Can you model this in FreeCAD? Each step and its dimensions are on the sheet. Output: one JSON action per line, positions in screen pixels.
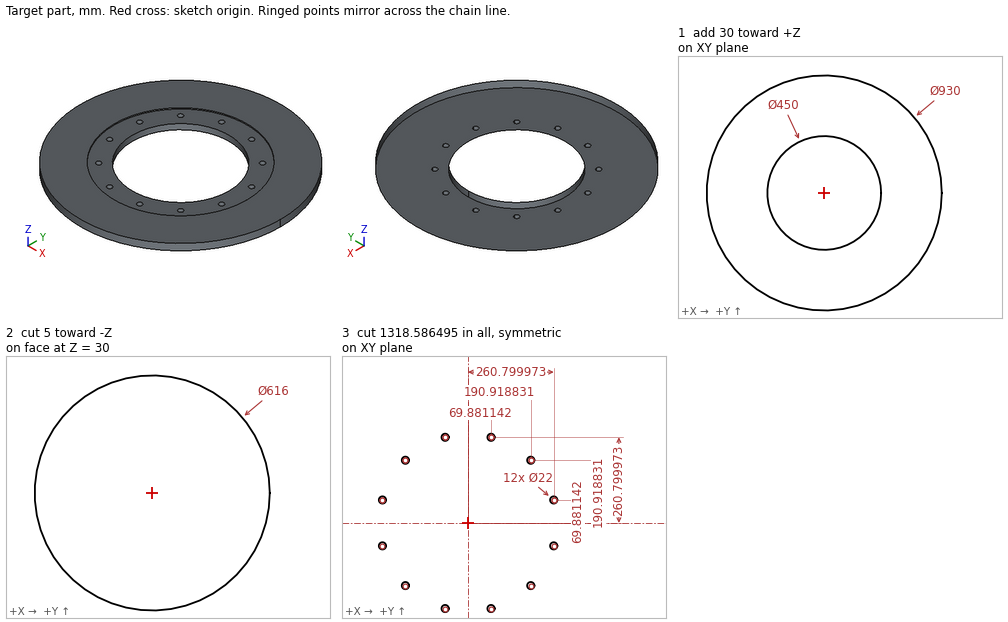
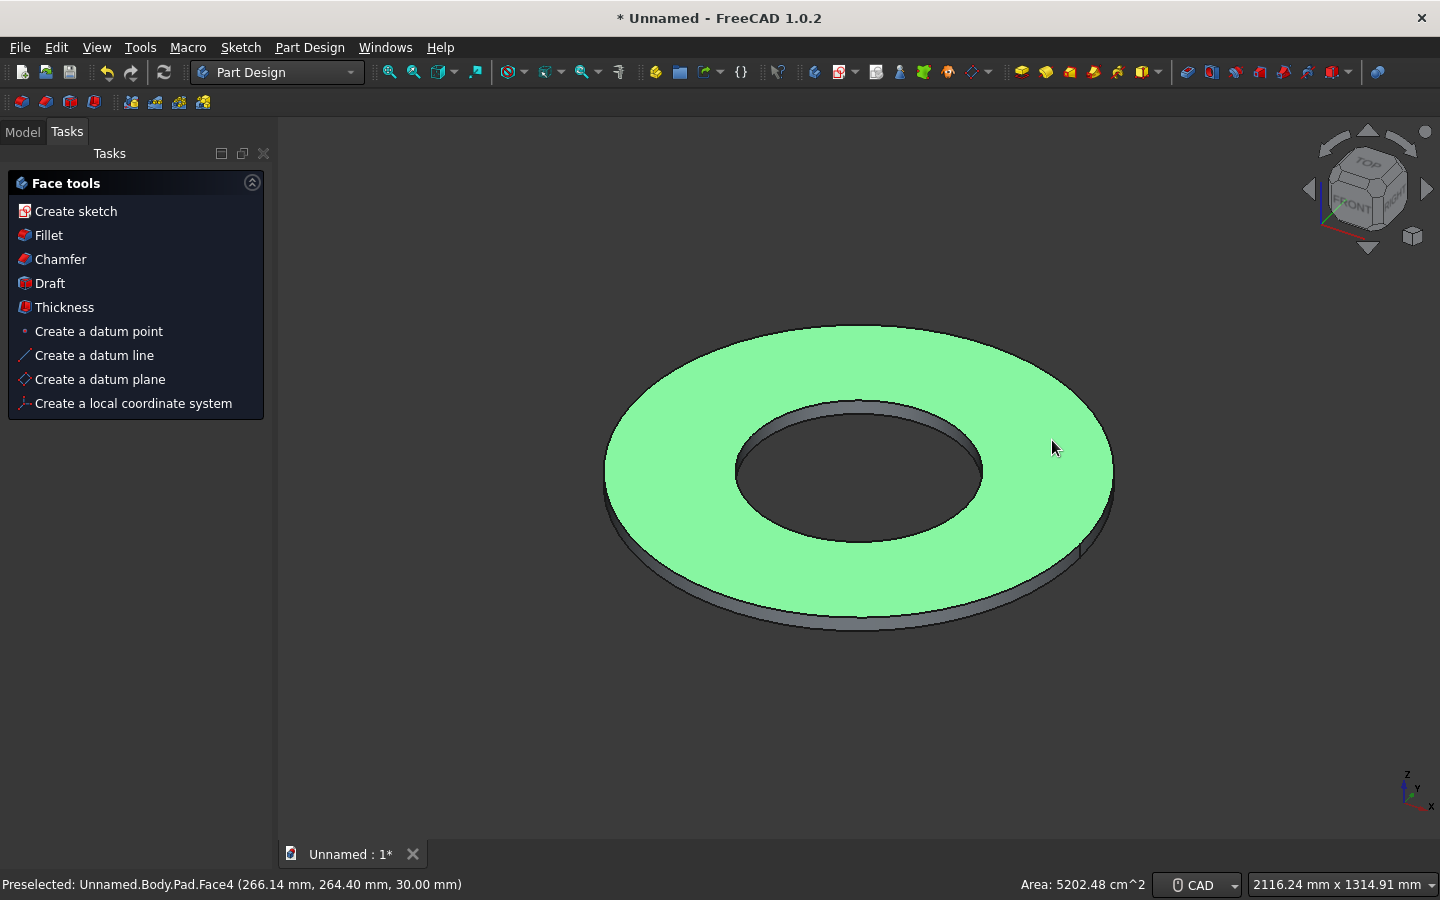
{"action": "left_click", "coordinate": [840, 72]}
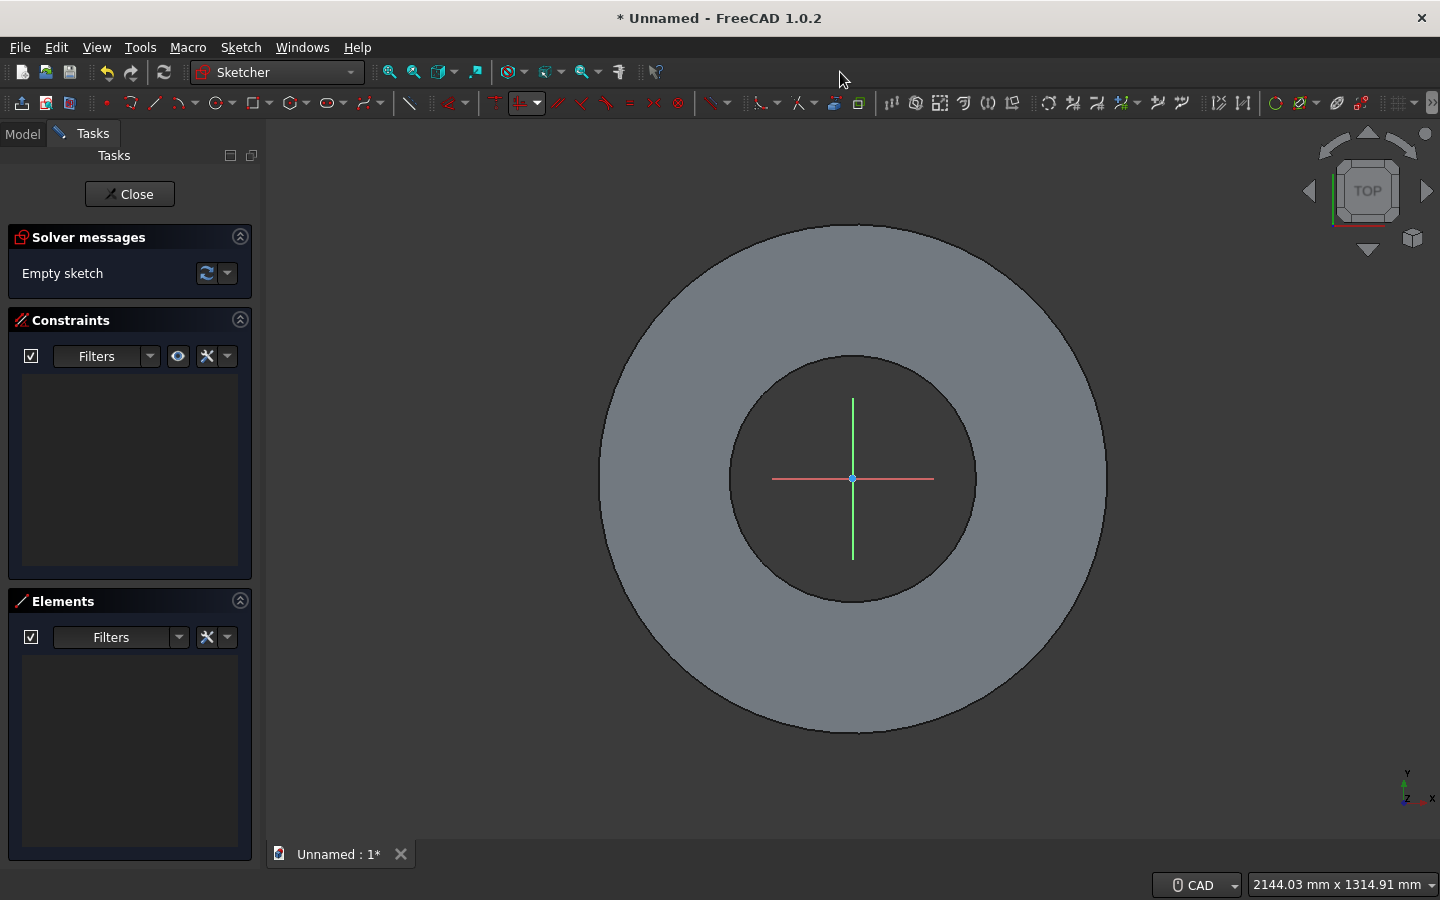
{"action": "scroll", "coordinate": [992, 479], "scroll_direction": "up", "scroll_amount": 2}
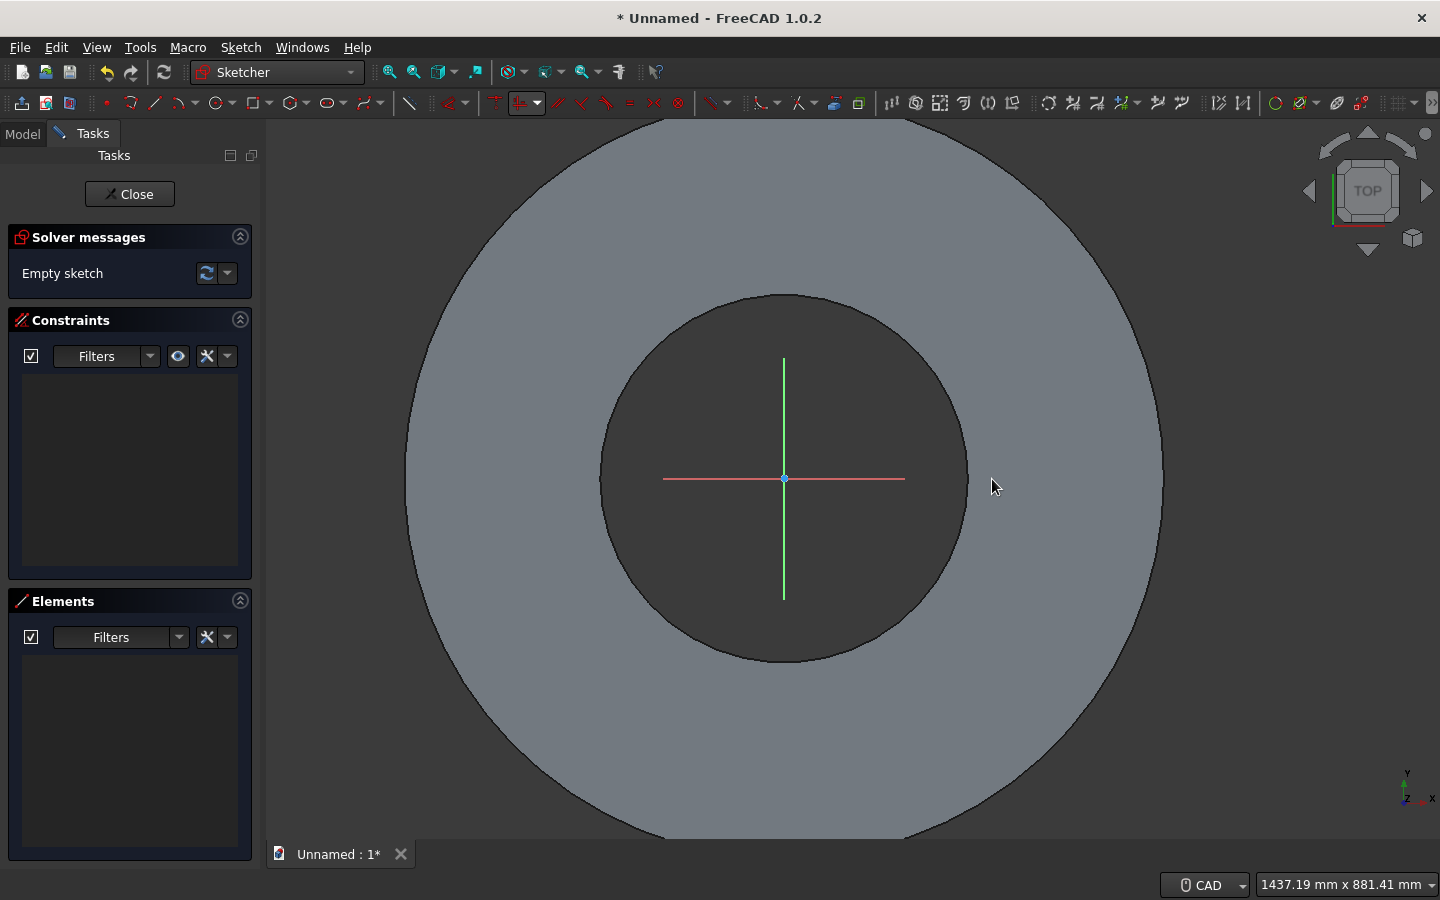
{"action": "left_click", "coordinate": [216, 104]}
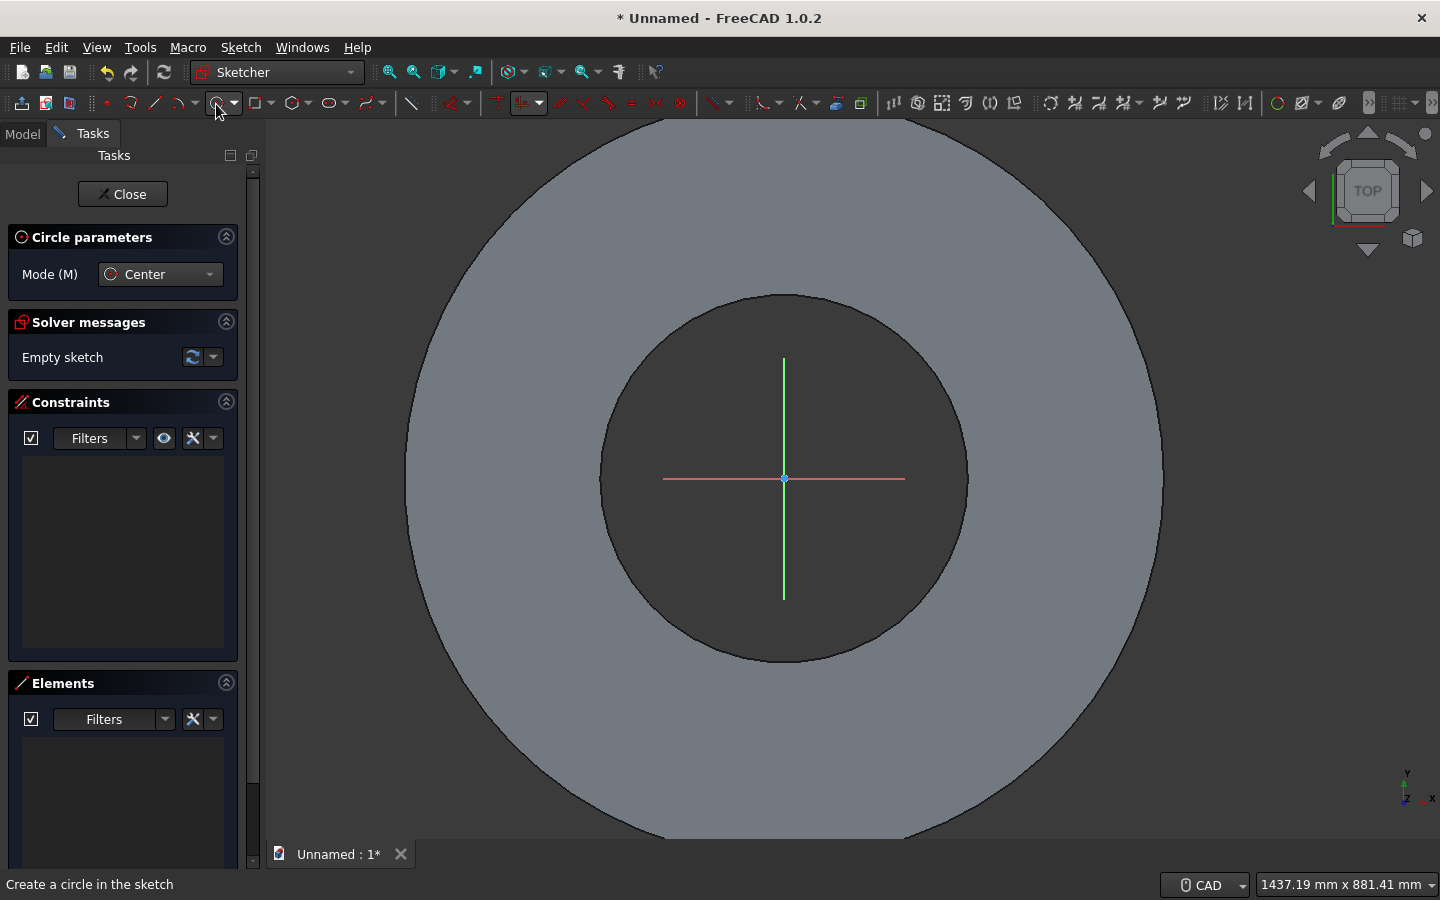
{"action": "left_click", "coordinate": [784, 479]}
{"action": "mouse_move", "coordinate": [962, 301]}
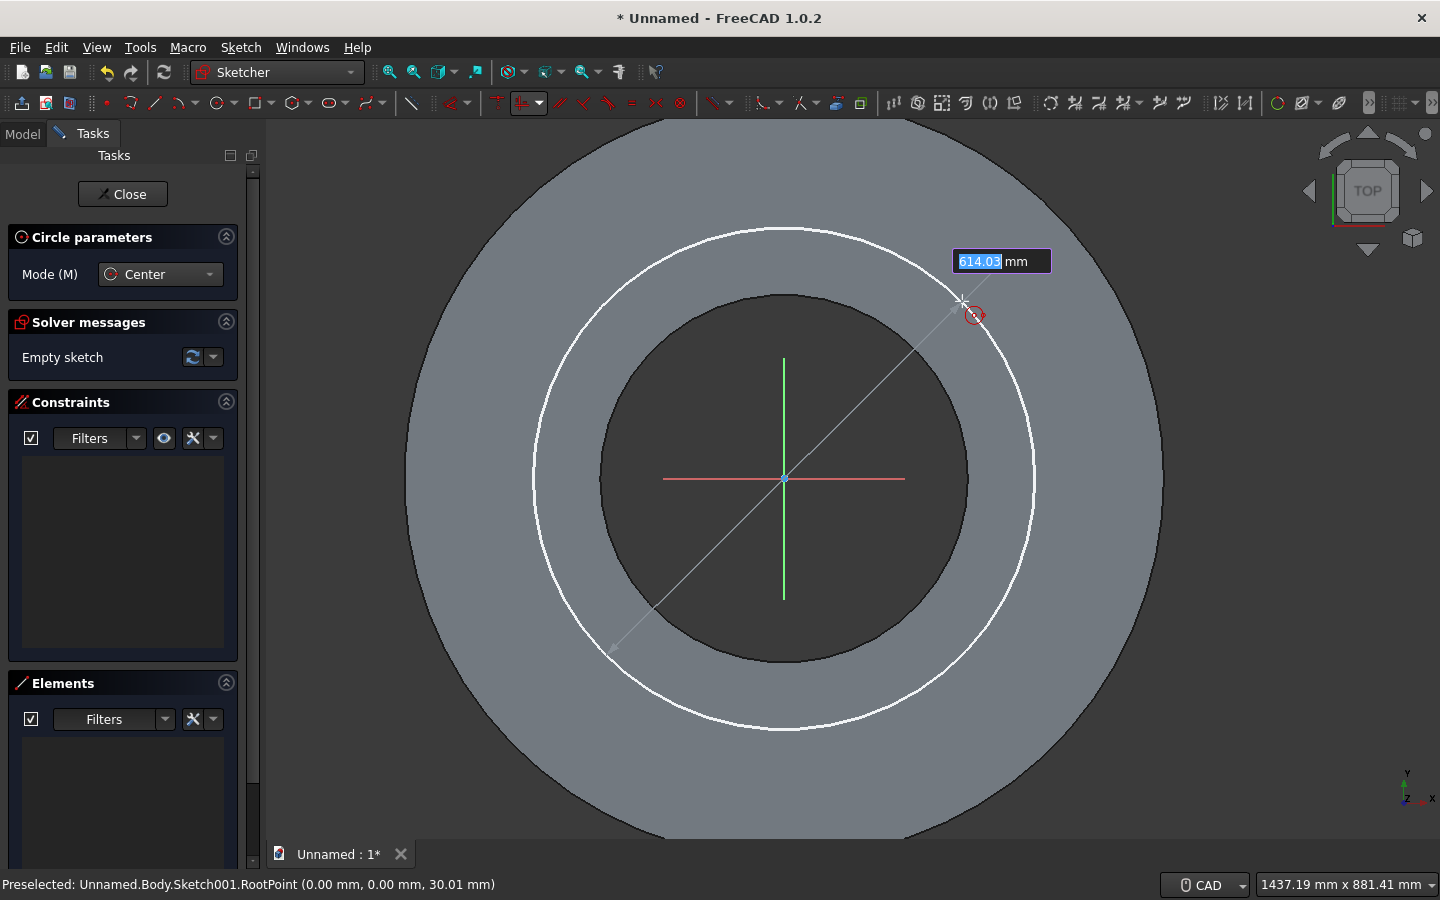
{"action": "type", "text": "616"}
{"action": "key", "text": "Return"}
{"action": "key", "text": "Escape"}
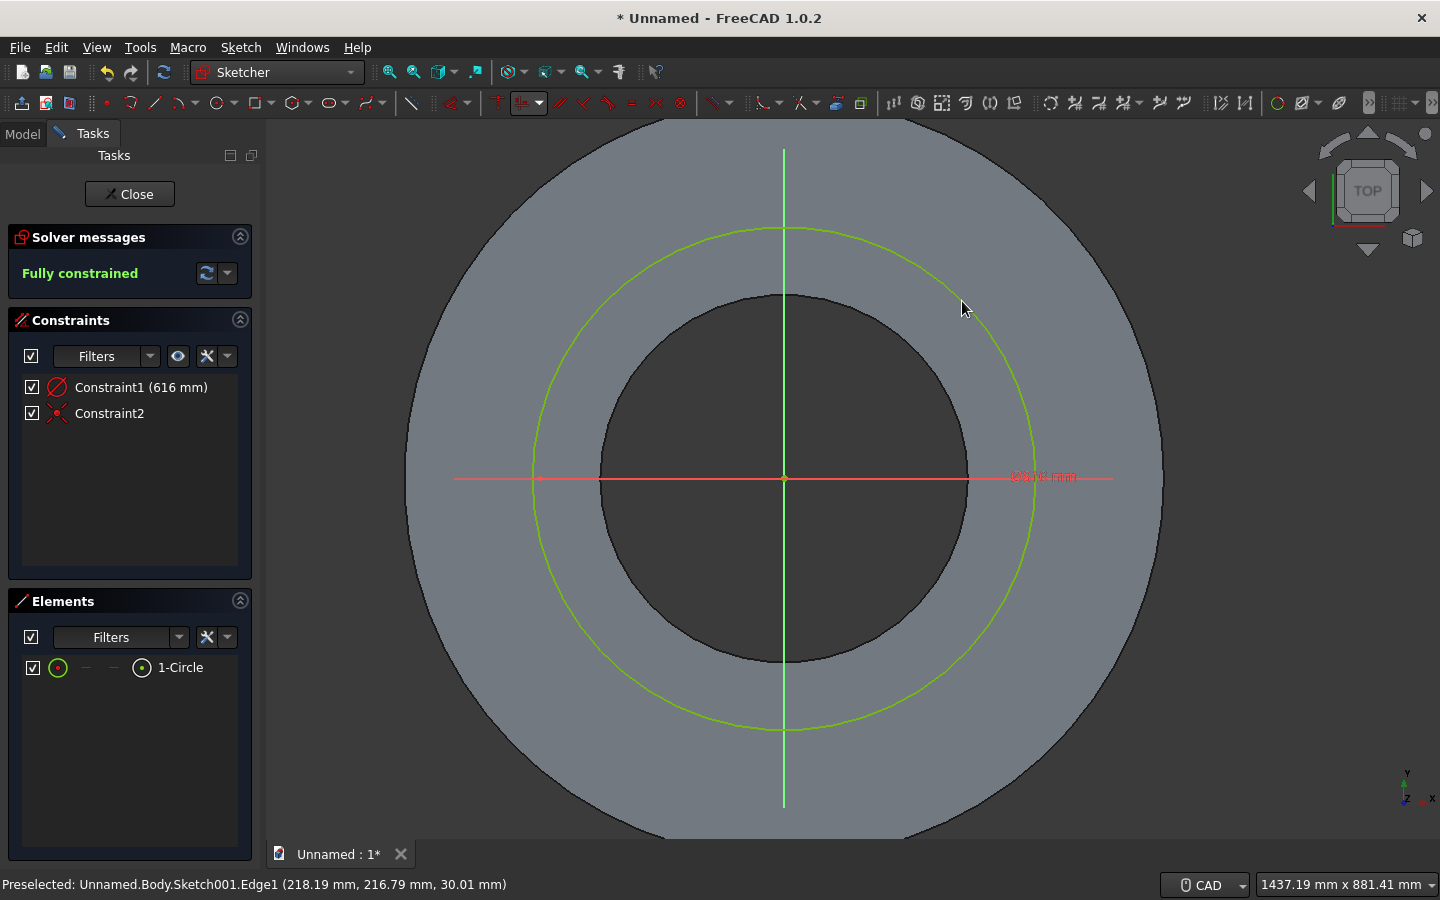
{"action": "left_click", "coordinate": [130, 194]}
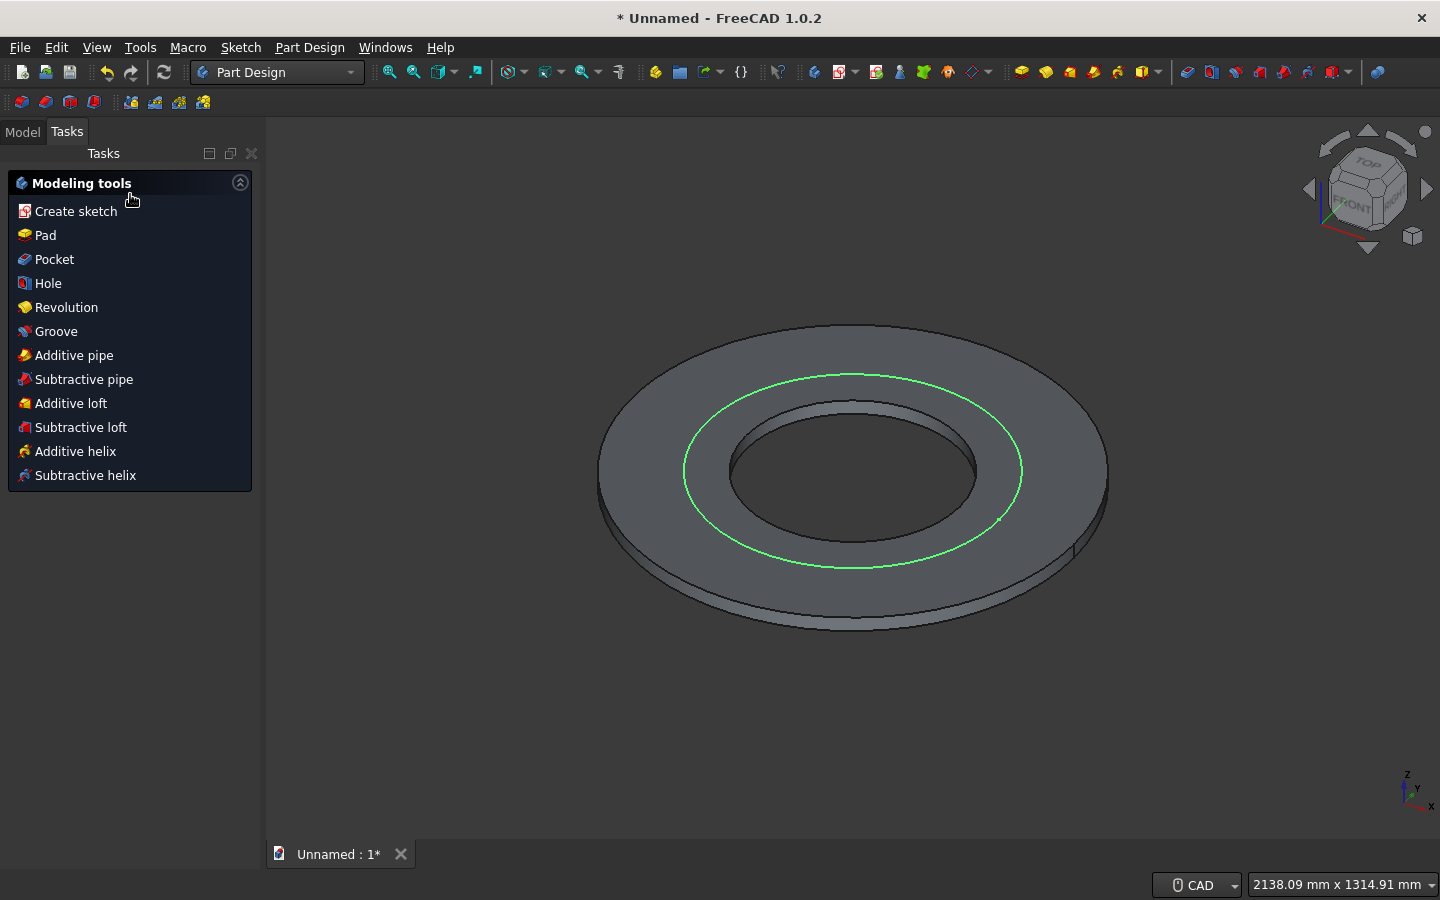
{"action": "left_click", "coordinate": [1188, 72]}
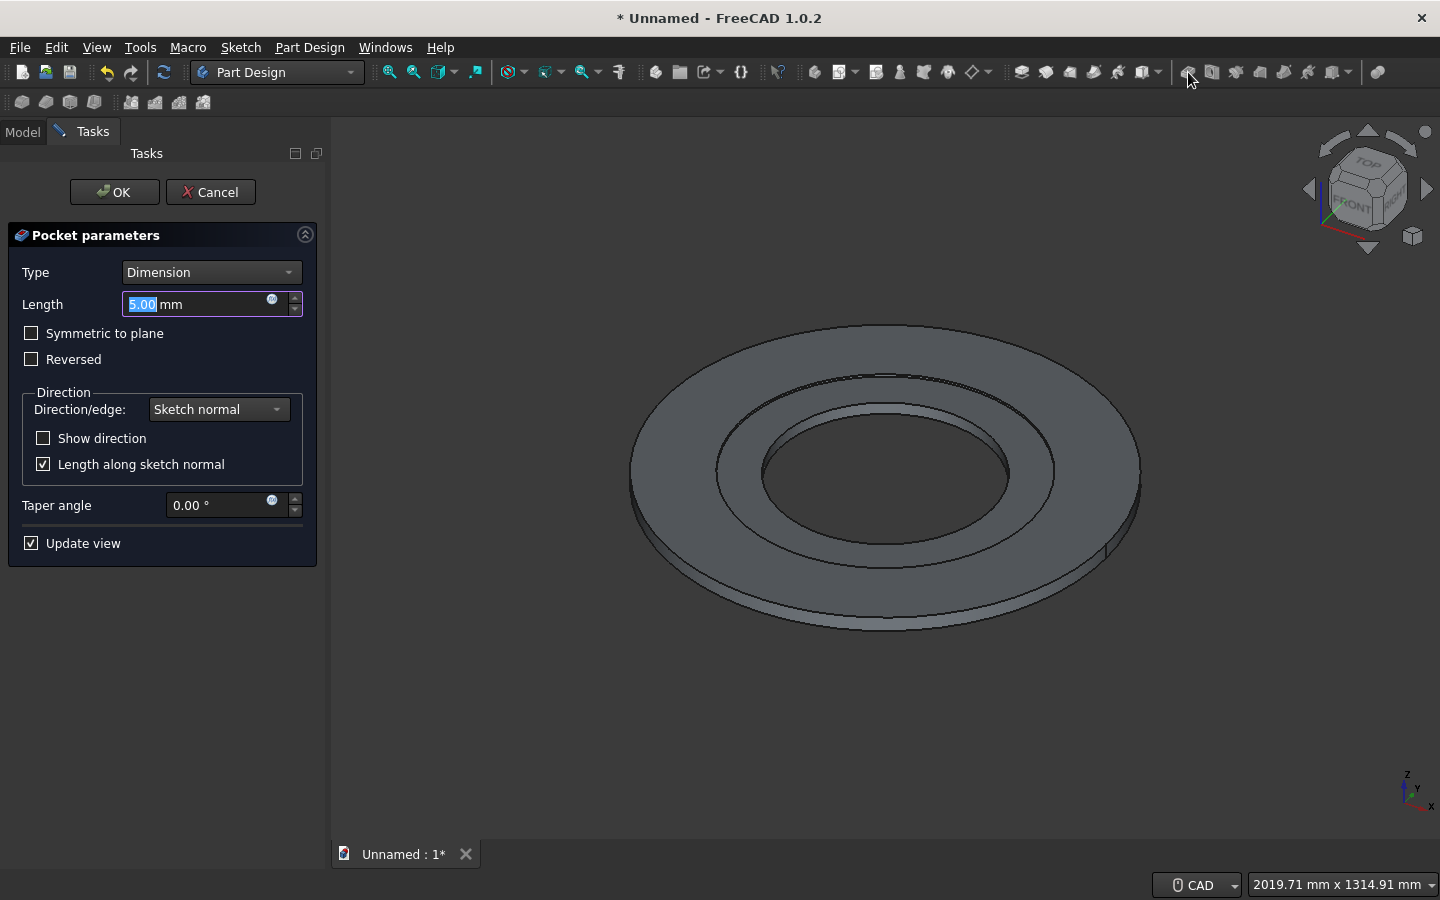
{"action": "type", "text": "5"}
{"action": "key", "text": "Tab"}